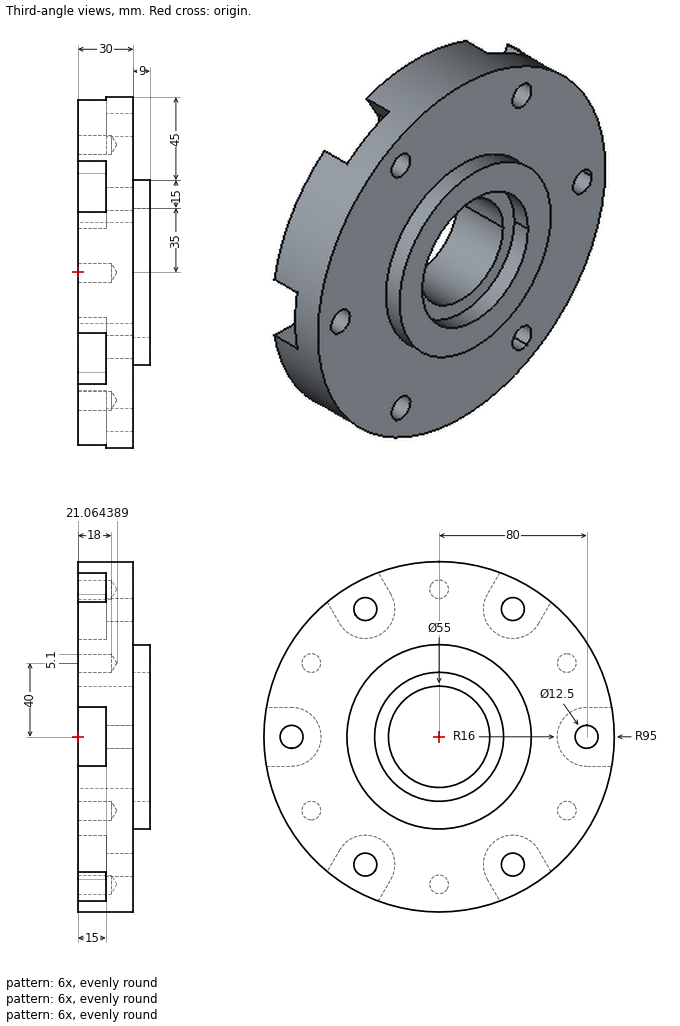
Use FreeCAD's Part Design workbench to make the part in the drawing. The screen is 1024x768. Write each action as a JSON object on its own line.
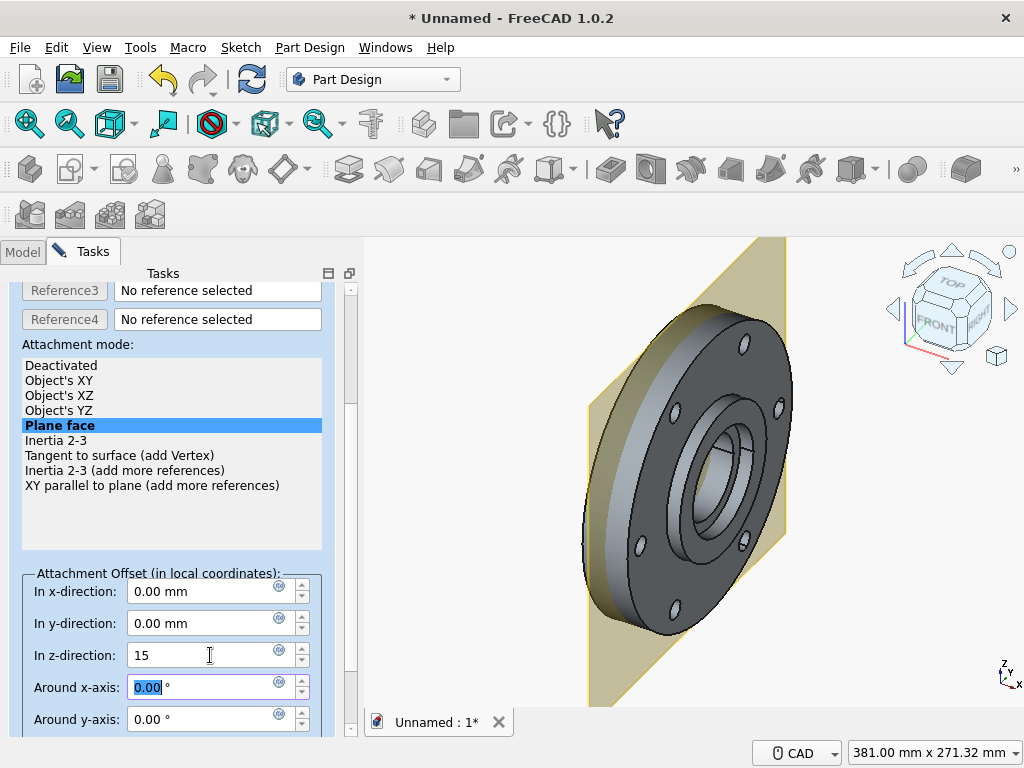
{"action": "scroll", "coordinate": [351, 510], "scroll_direction": "up", "scroll_amount": 4}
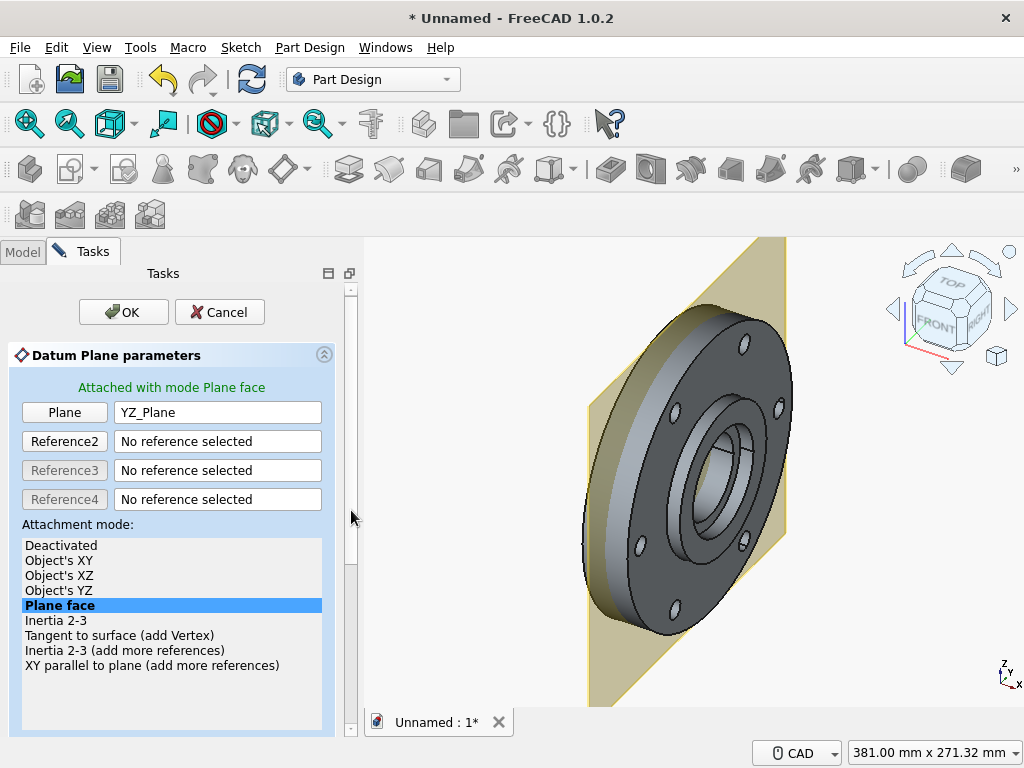
{"action": "left_click", "coordinate": [124, 312]}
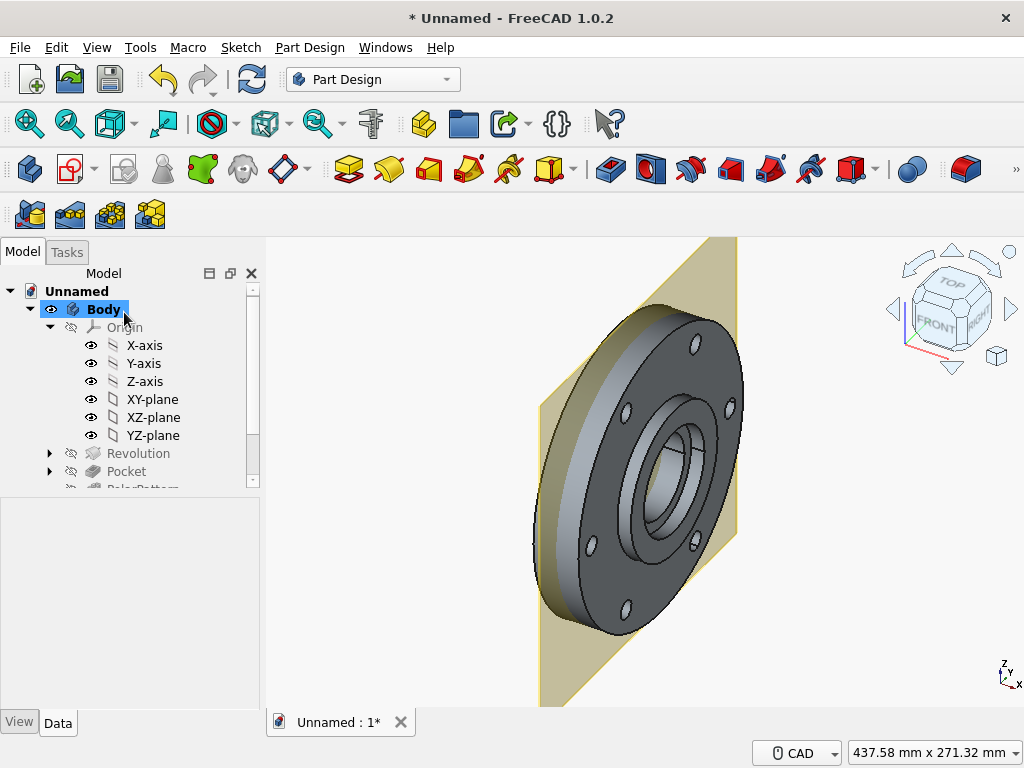
{"action": "scroll", "coordinate": [100, 377], "scroll_direction": "down", "scroll_amount": 3}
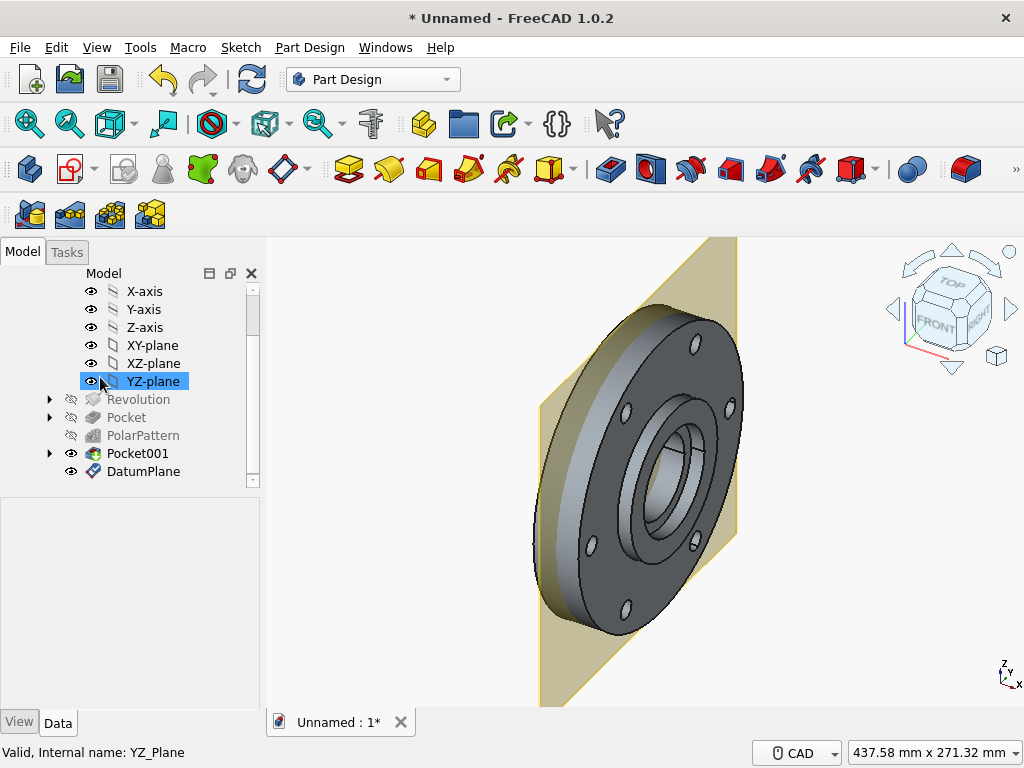
{"action": "left_click", "coordinate": [116, 471]}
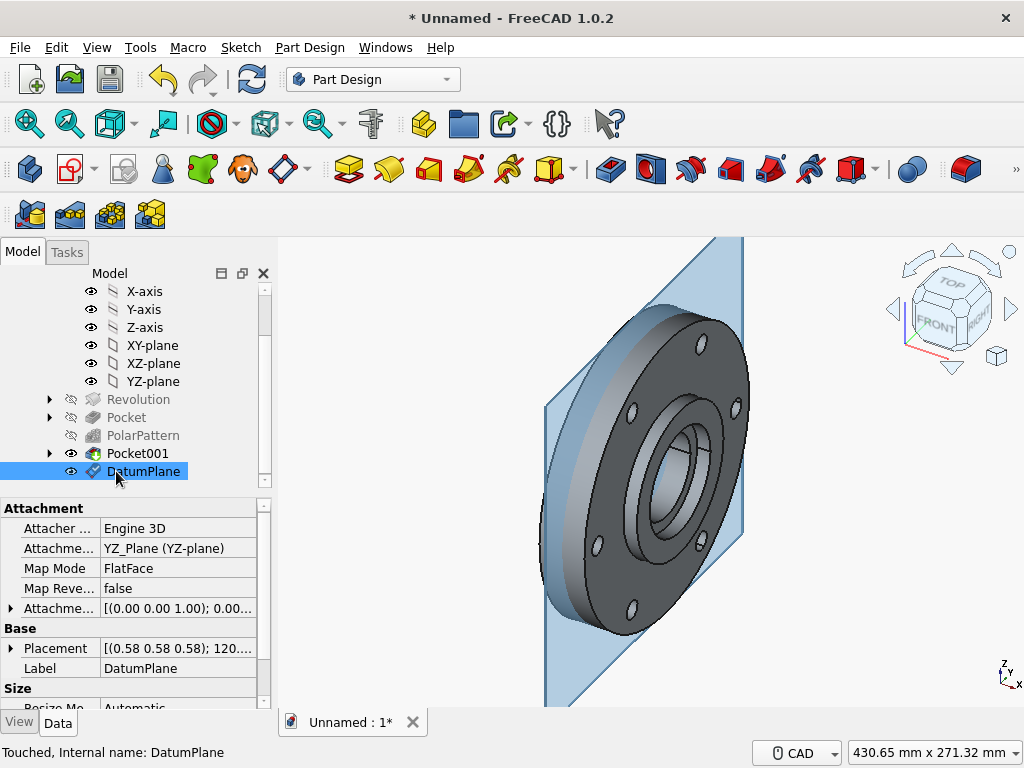
{"action": "left_click", "coordinate": [70, 170]}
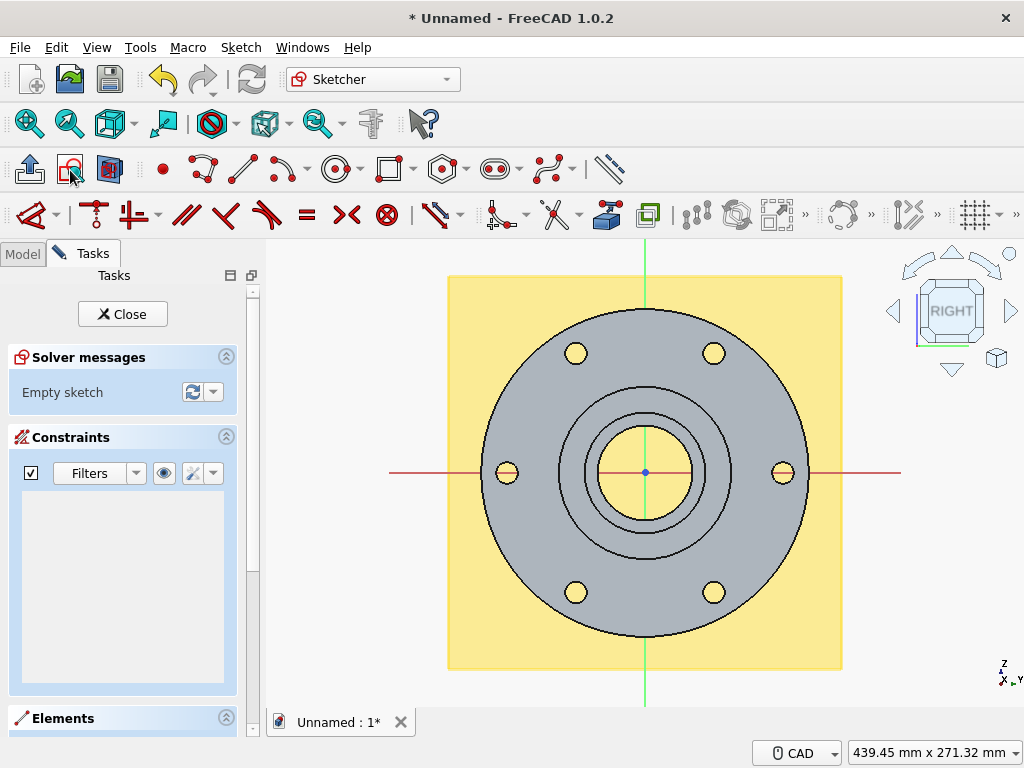
{"action": "left_click", "coordinate": [110, 170]}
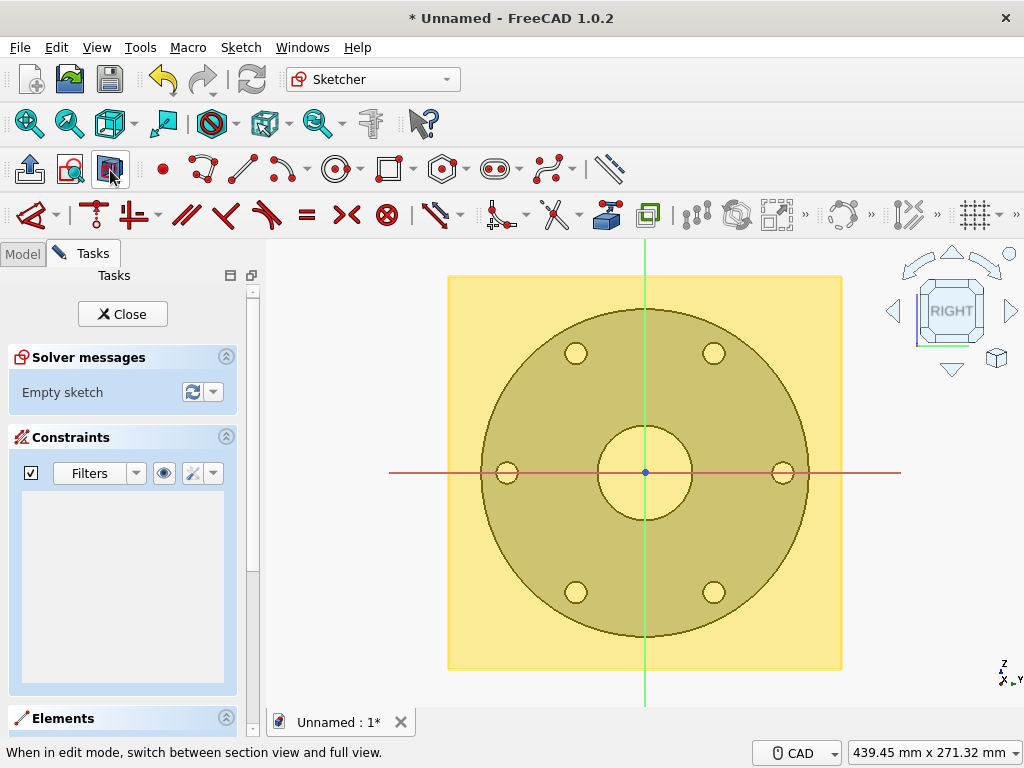
{"action": "scroll", "coordinate": [834, 473], "scroll_direction": "up", "scroll_amount": 8}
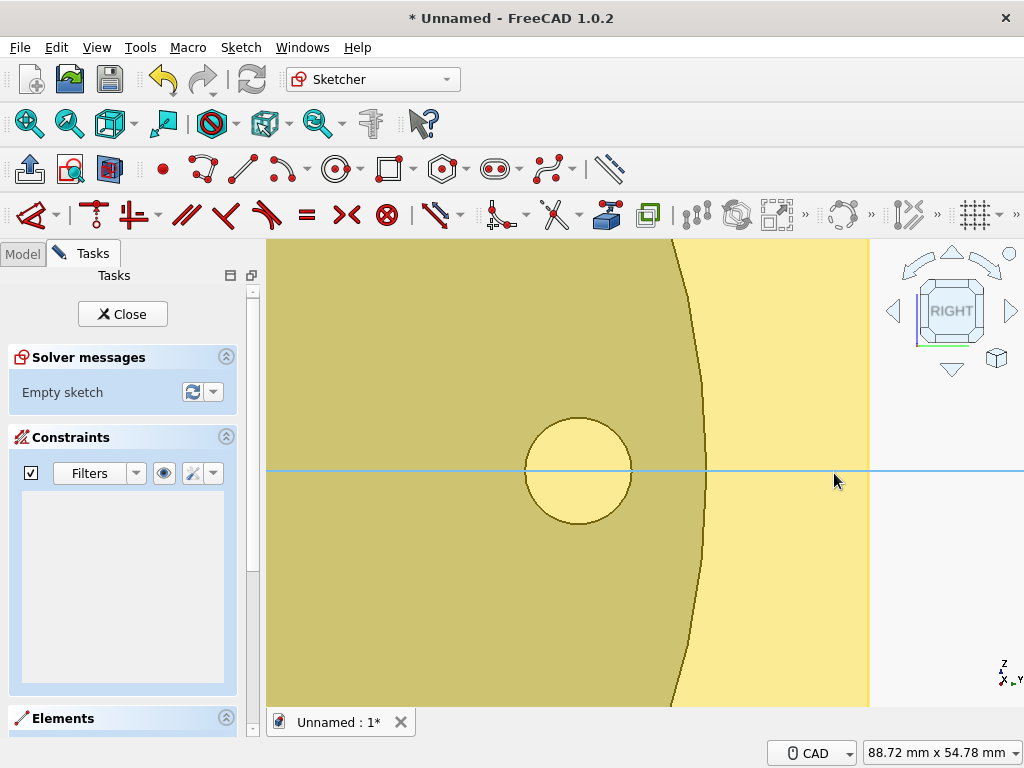
{"action": "left_click", "coordinate": [244, 170]}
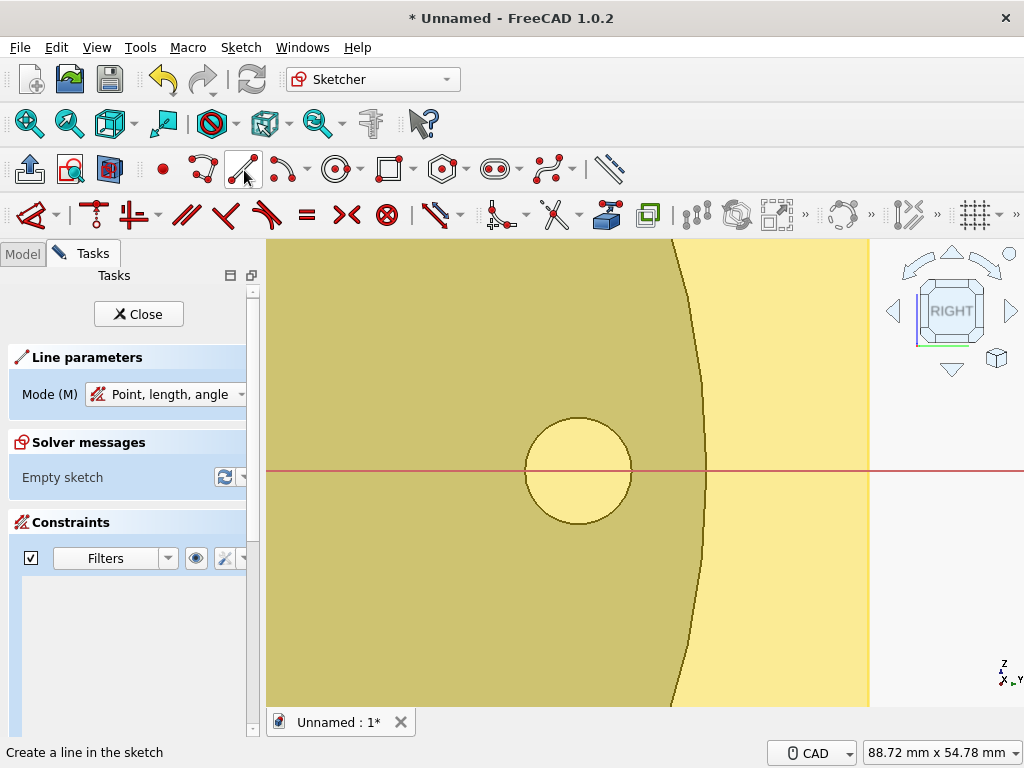
{"action": "left_click", "coordinate": [695, 608]}
{"action": "left_click", "coordinate": [578, 608]}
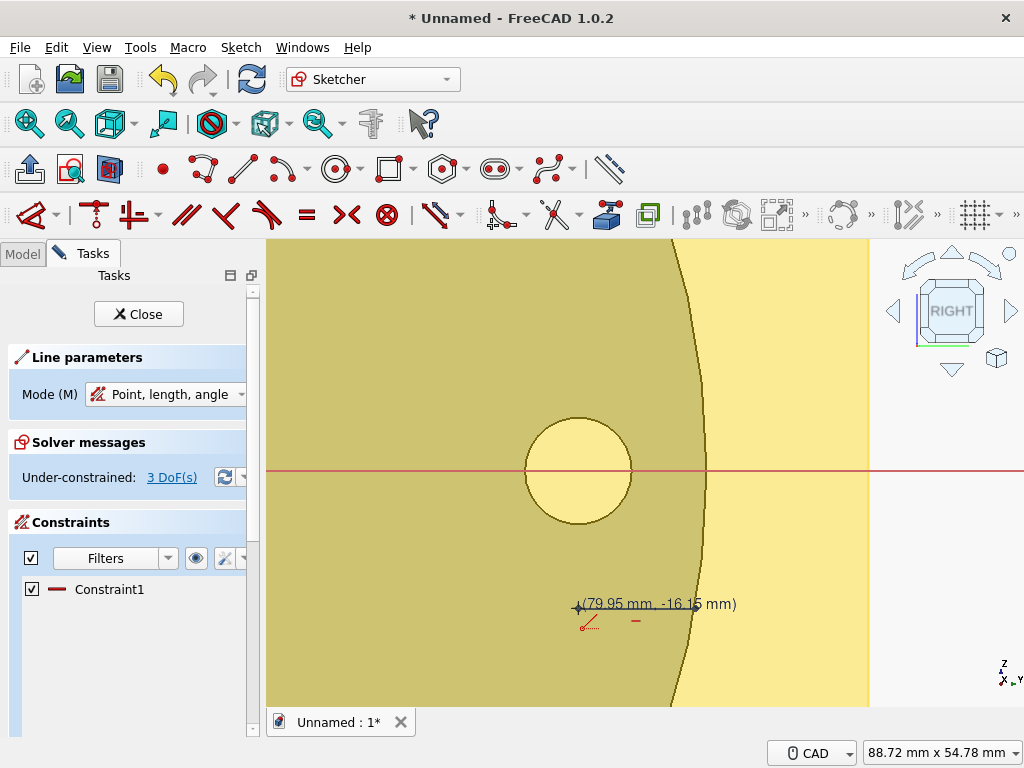
{"action": "left_click", "coordinate": [578, 334]}
{"action": "left_click", "coordinate": [695, 334]}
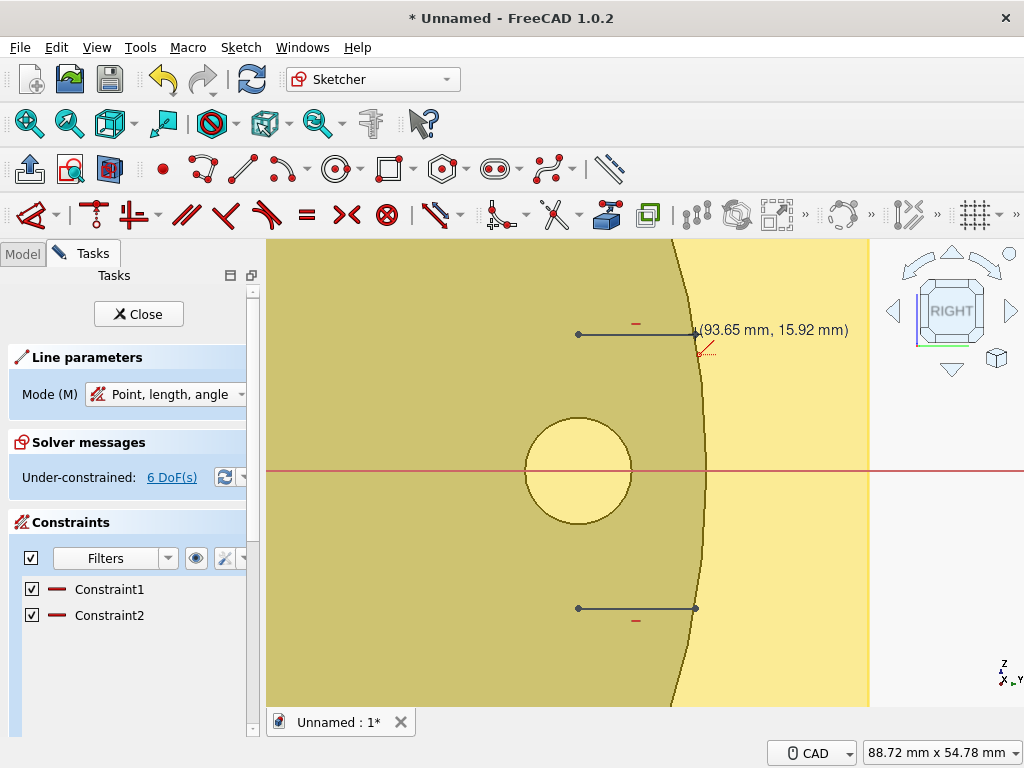
{"action": "key", "text": "g 3 a"}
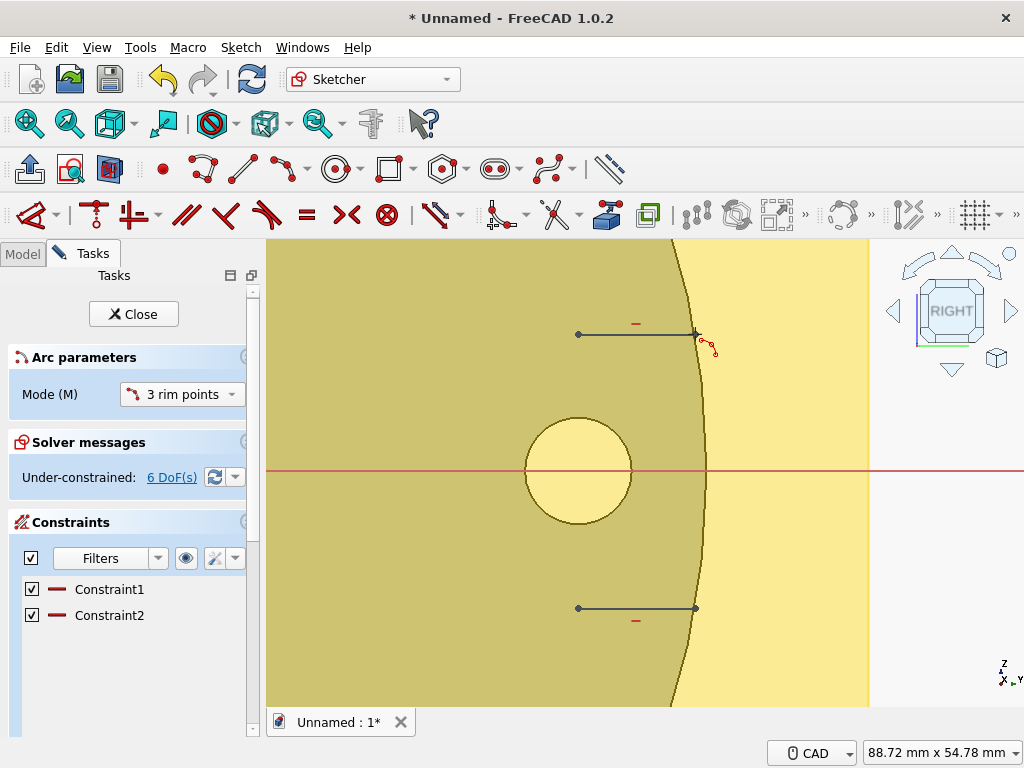
{"action": "left_click", "coordinate": [578, 609]}
{"action": "left_click", "coordinate": [578, 335]}
{"action": "left_click", "coordinate": [448, 429]}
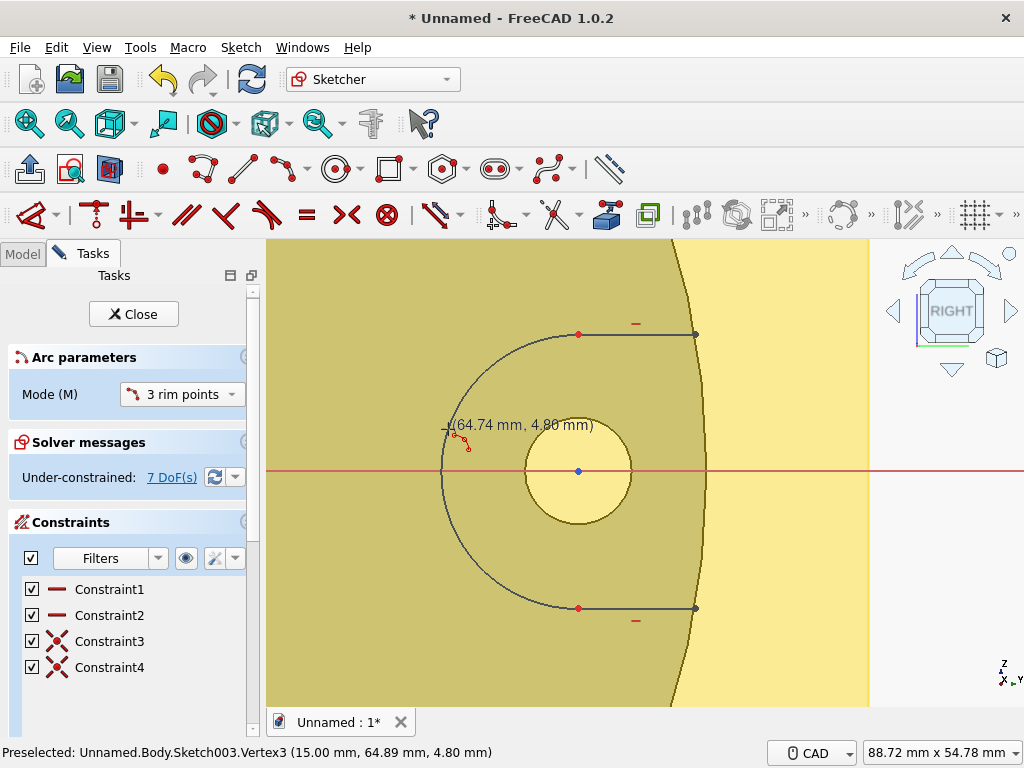
{"action": "left_click", "coordinate": [695, 335]}
{"action": "left_click", "coordinate": [695, 609]}